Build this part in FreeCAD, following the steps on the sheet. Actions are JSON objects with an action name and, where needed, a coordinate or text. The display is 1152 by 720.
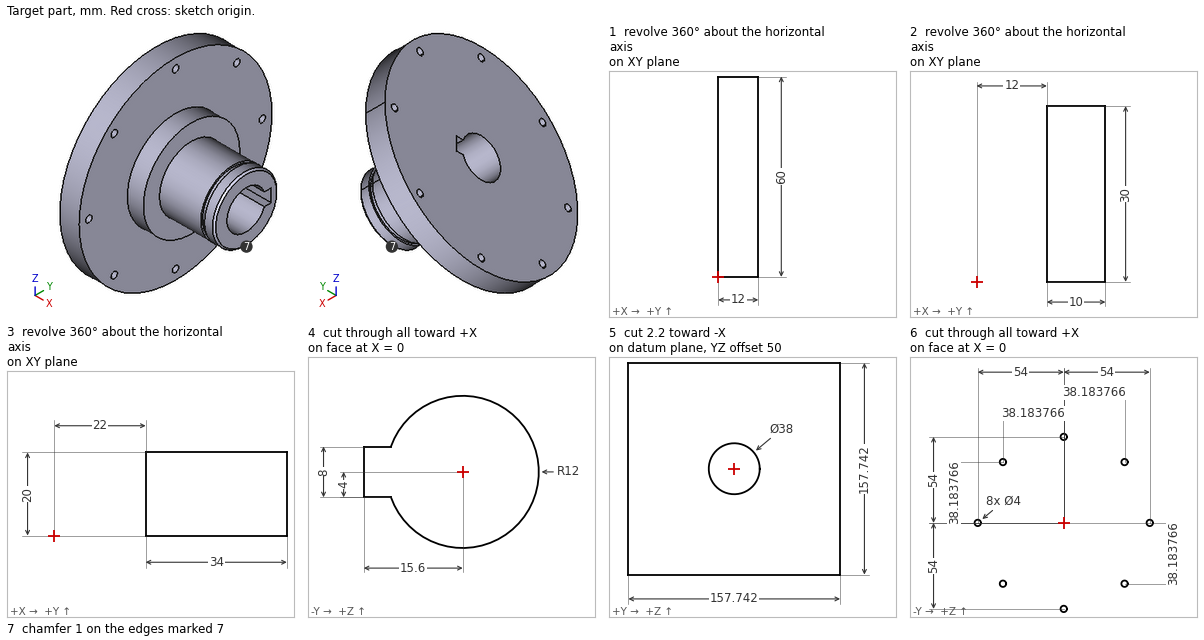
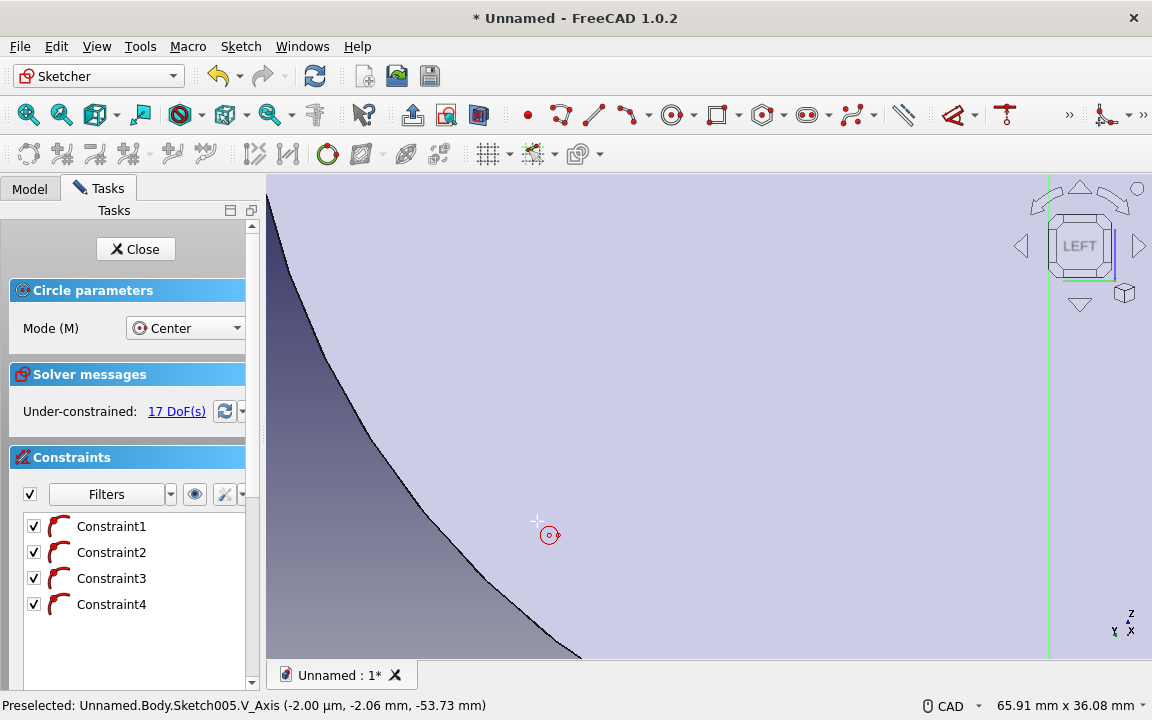
{"action": "scroll", "coordinate": [537, 521], "scroll_direction": "down", "scroll_amount": 8}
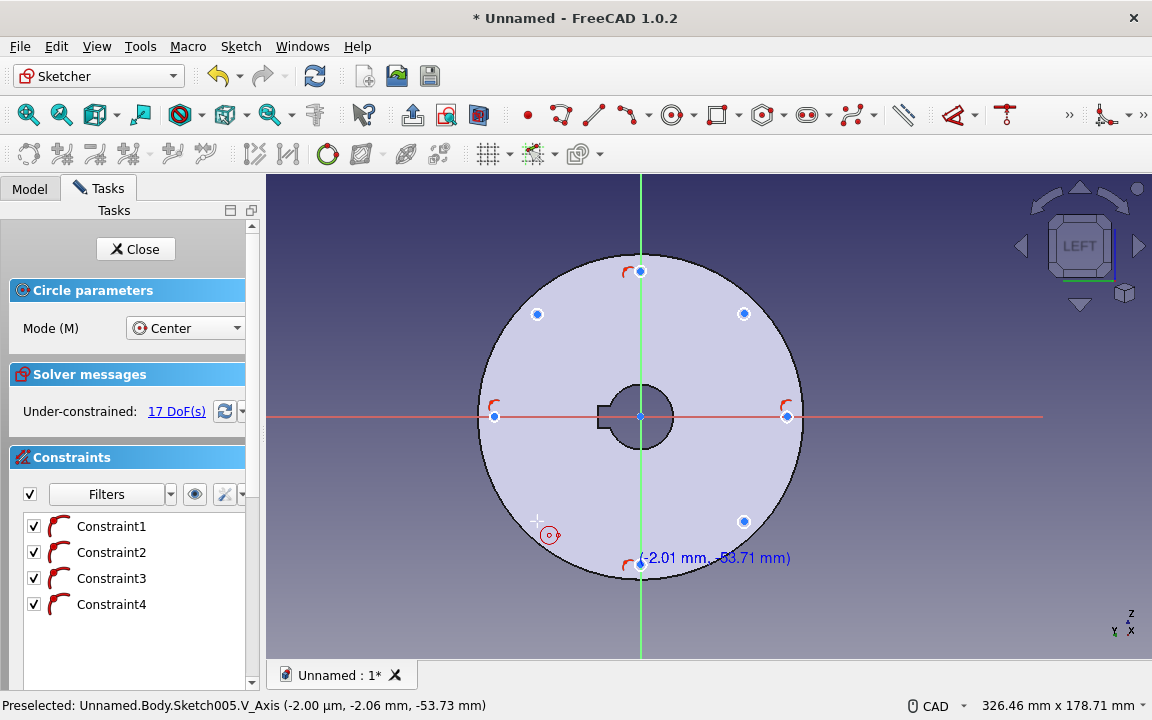
{"action": "left_click", "coordinate": [537, 521]}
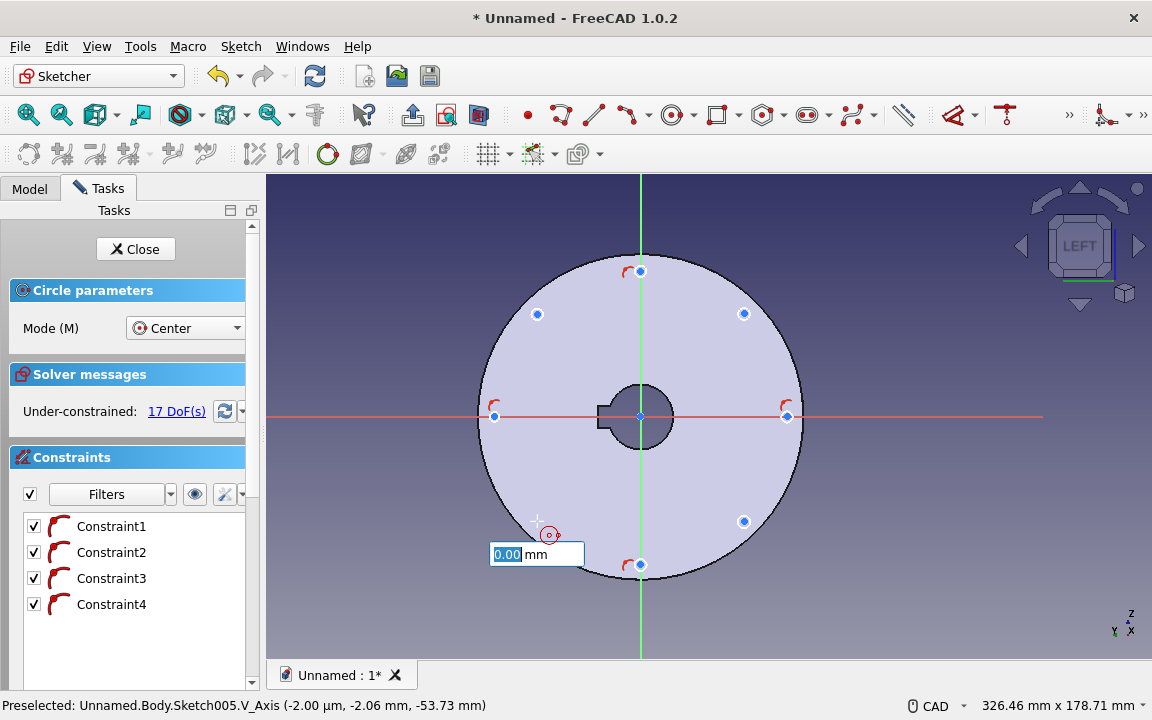
{"action": "scroll", "coordinate": [541, 517], "scroll_direction": "up", "scroll_amount": 6}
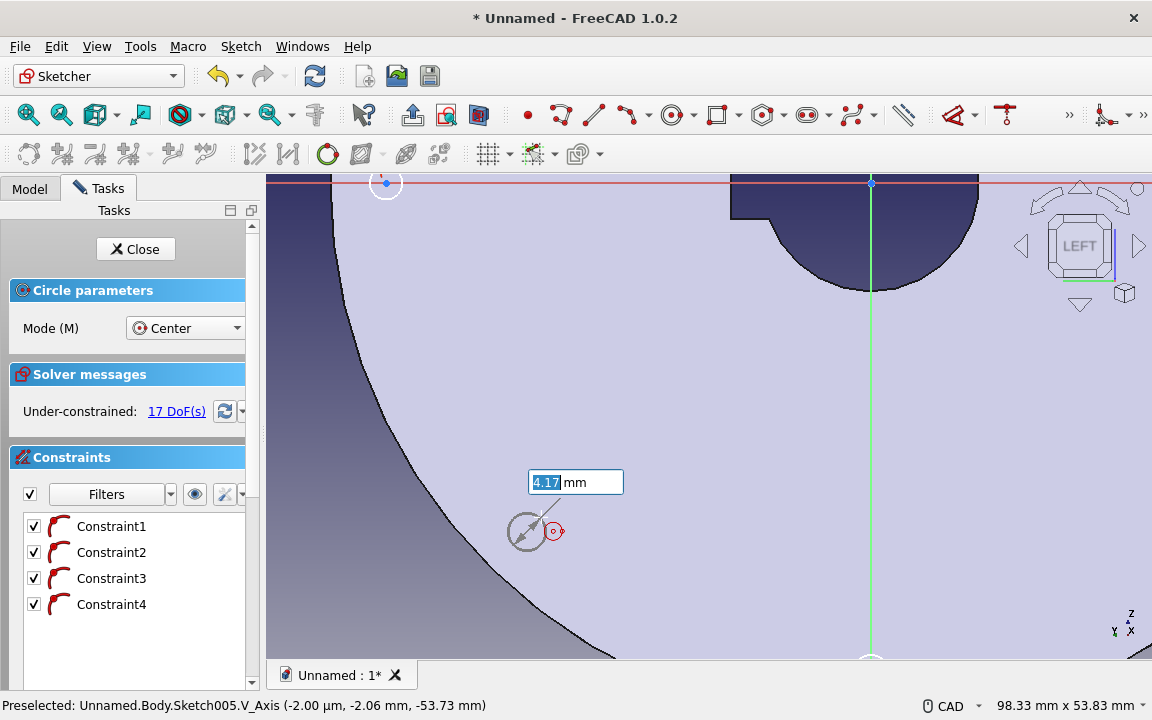
{"action": "left_click", "coordinate": [540, 515]}
{"action": "key", "text": "Escape"}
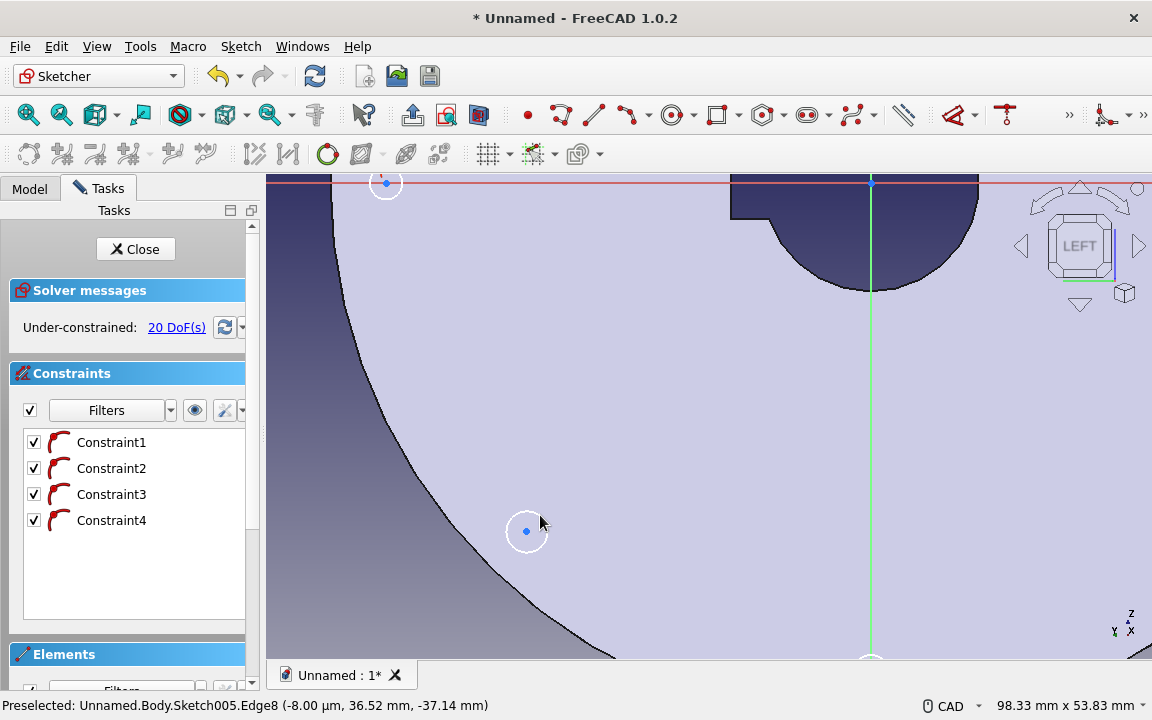
{"action": "scroll", "coordinate": [541, 517], "scroll_direction": "down", "scroll_amount": 6}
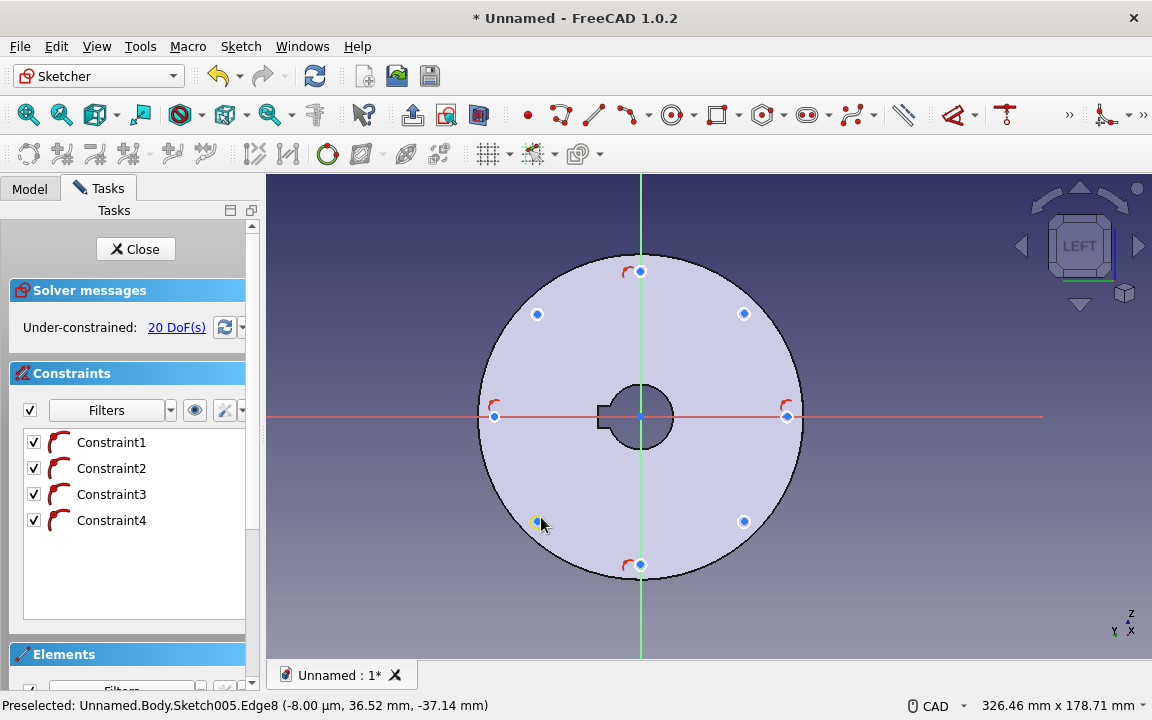
{"action": "scroll", "coordinate": [498, 414], "scroll_direction": "up", "scroll_amount": 7}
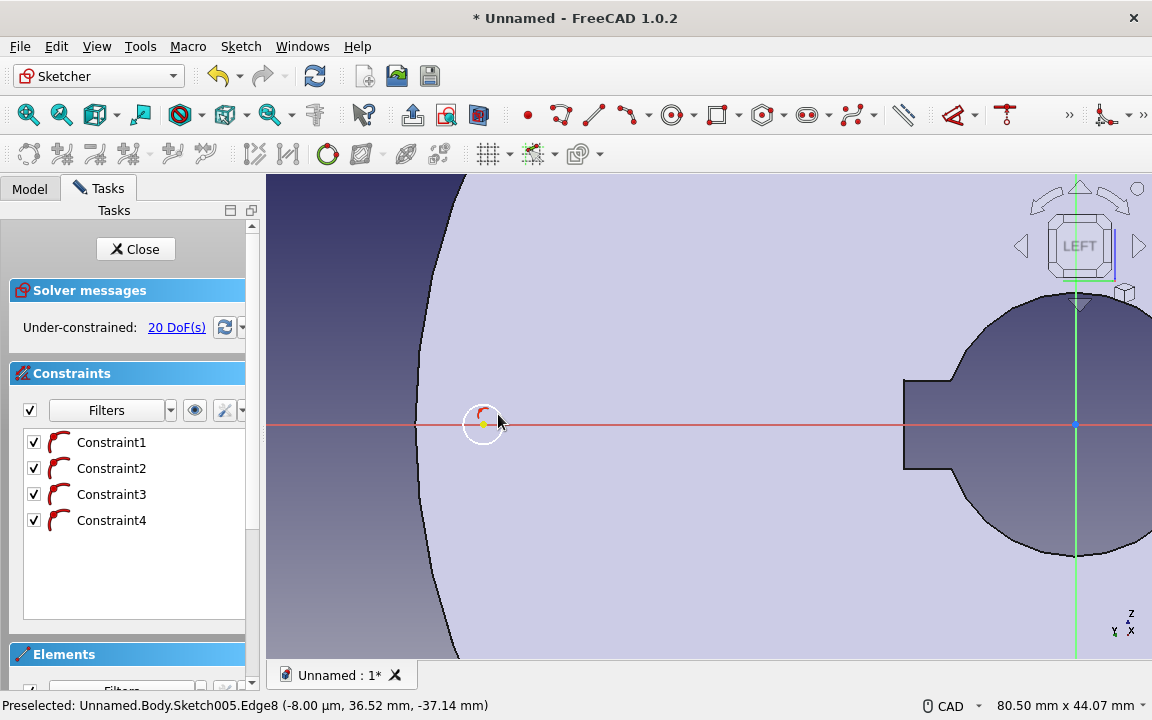
{"action": "left_click", "coordinate": [497, 410]}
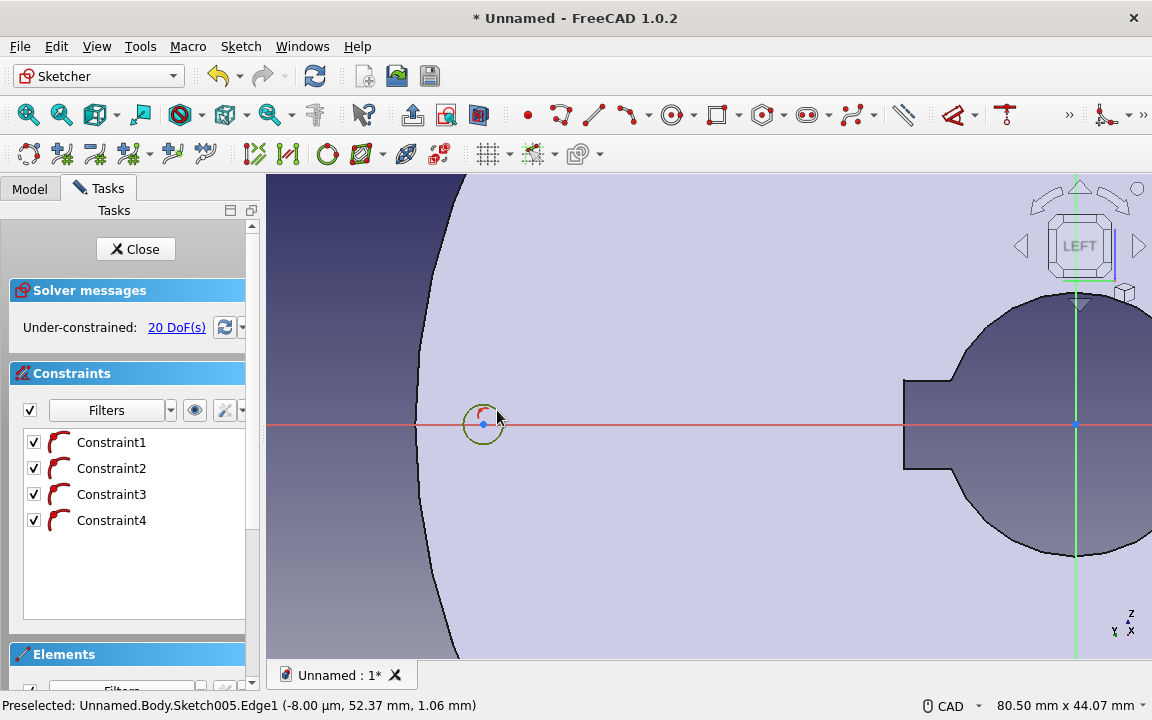
{"action": "scroll", "coordinate": [498, 414], "scroll_direction": "down", "scroll_amount": 7}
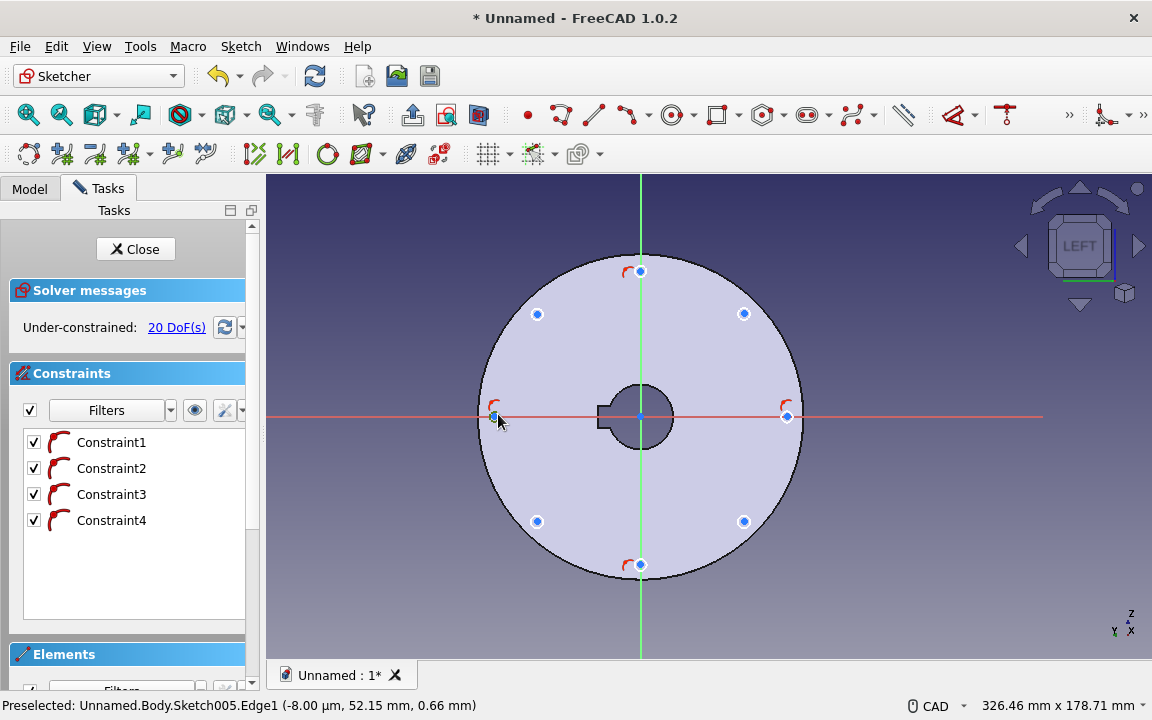
{"action": "scroll", "coordinate": [541, 310], "scroll_direction": "up", "scroll_amount": 5}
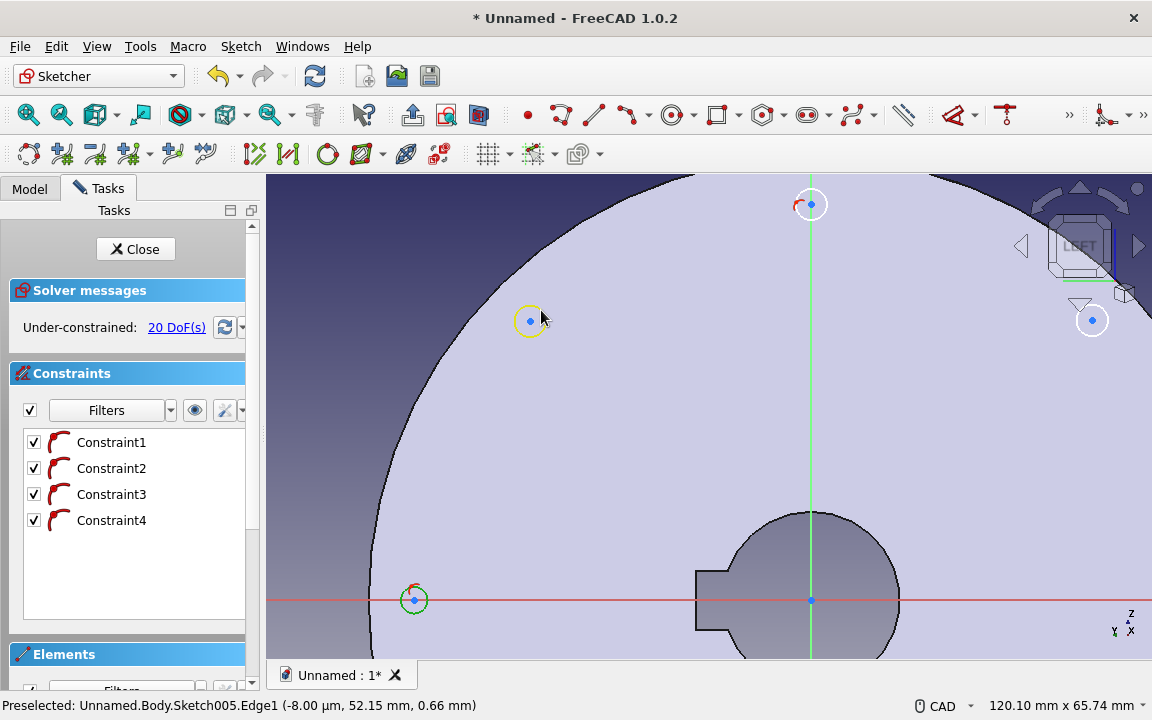
{"action": "left_click", "coordinate": [541, 310]}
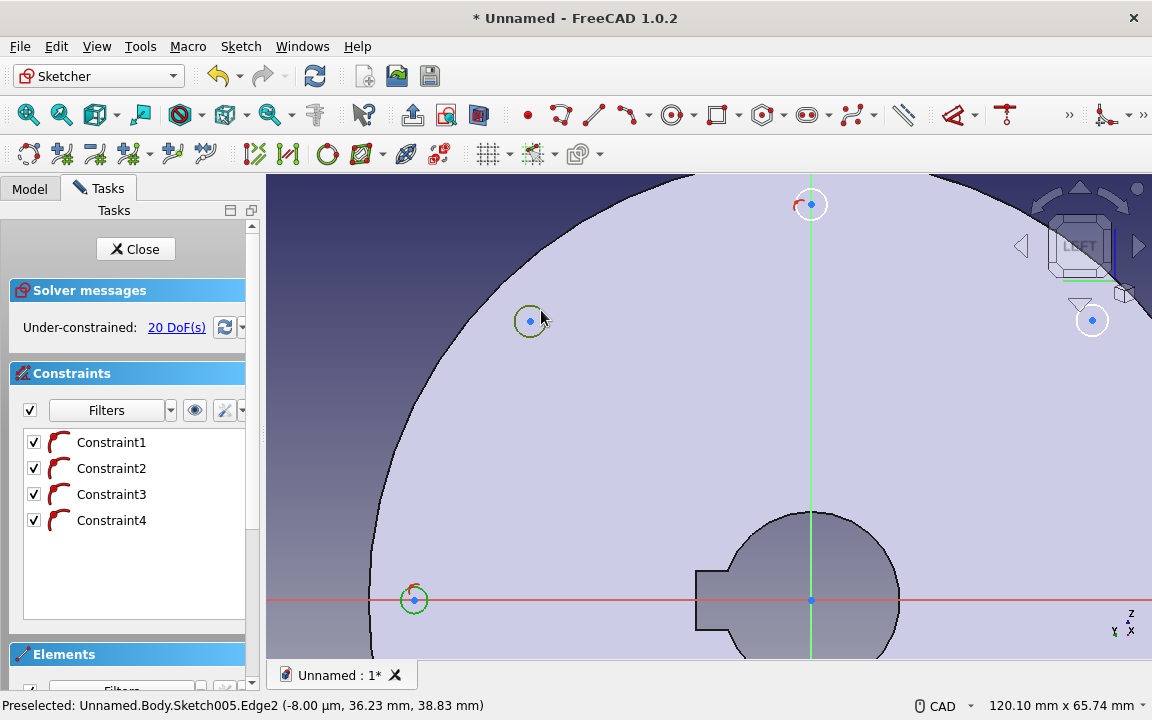
{"action": "scroll", "coordinate": [800, 216], "scroll_direction": "up", "scroll_amount": 2}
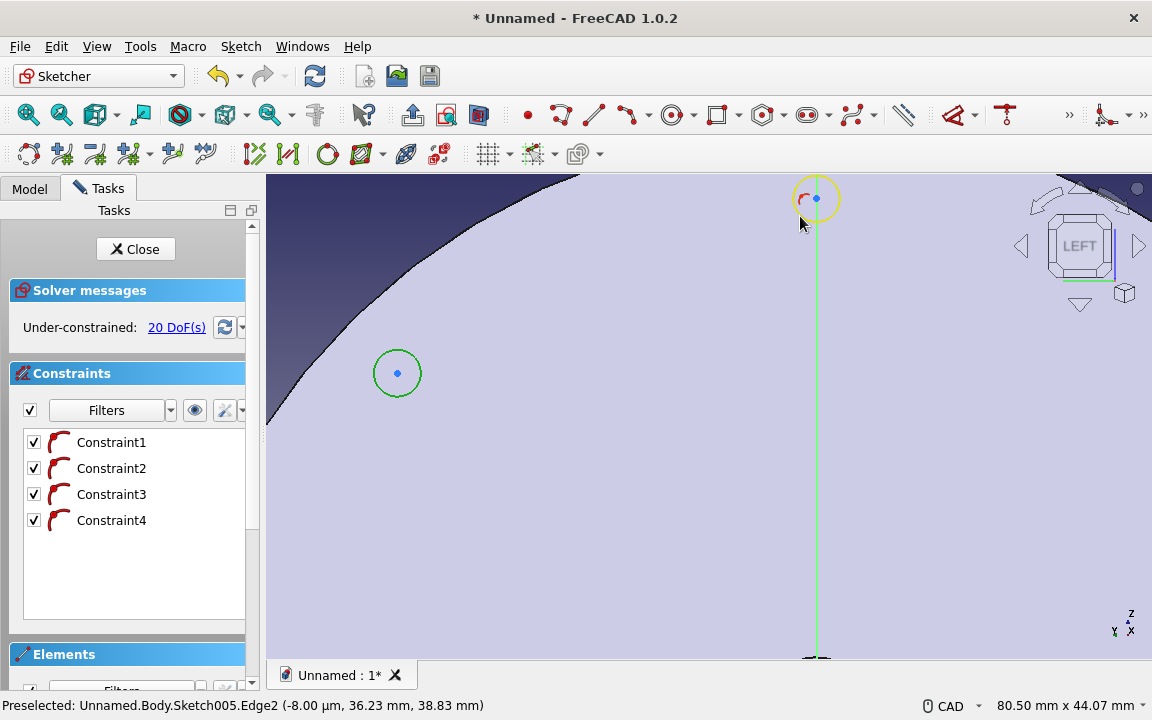
{"action": "left_click", "coordinate": [800, 215]}